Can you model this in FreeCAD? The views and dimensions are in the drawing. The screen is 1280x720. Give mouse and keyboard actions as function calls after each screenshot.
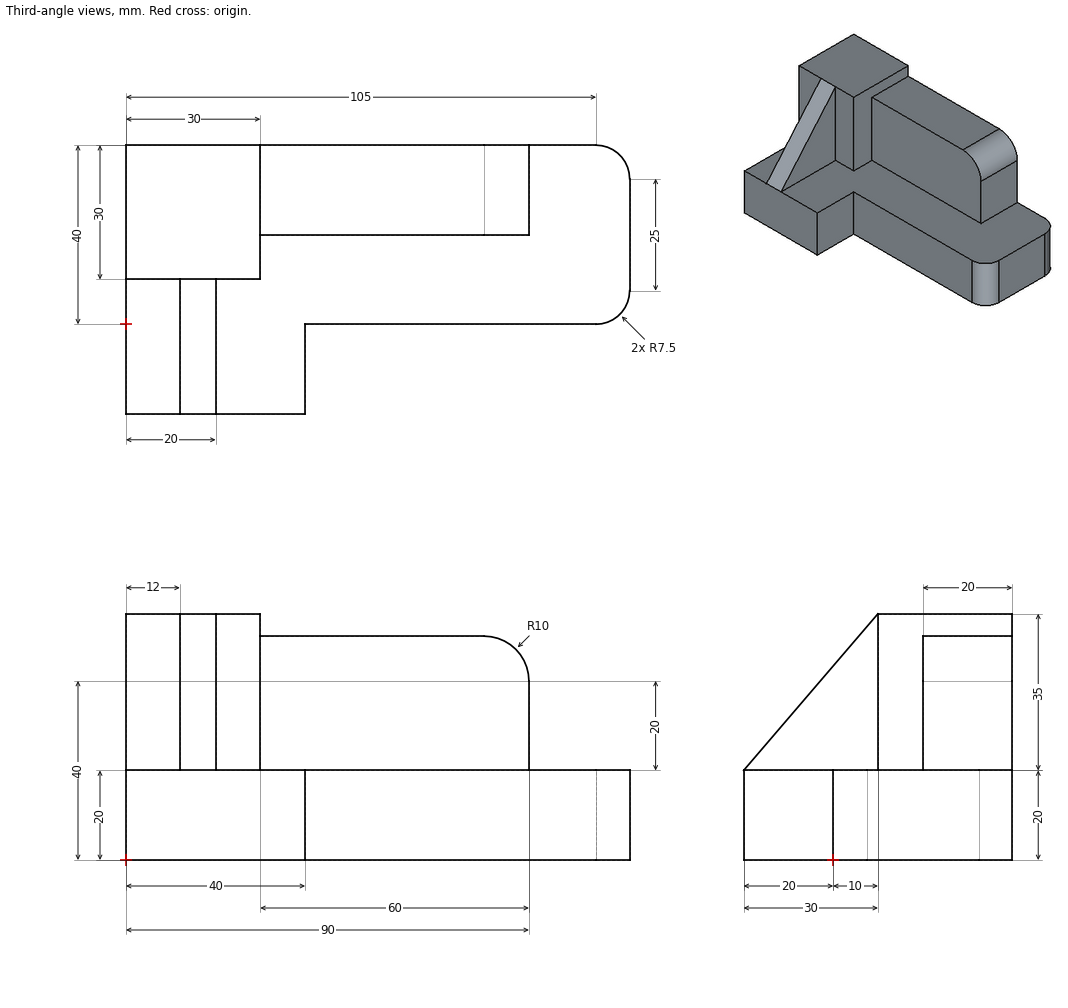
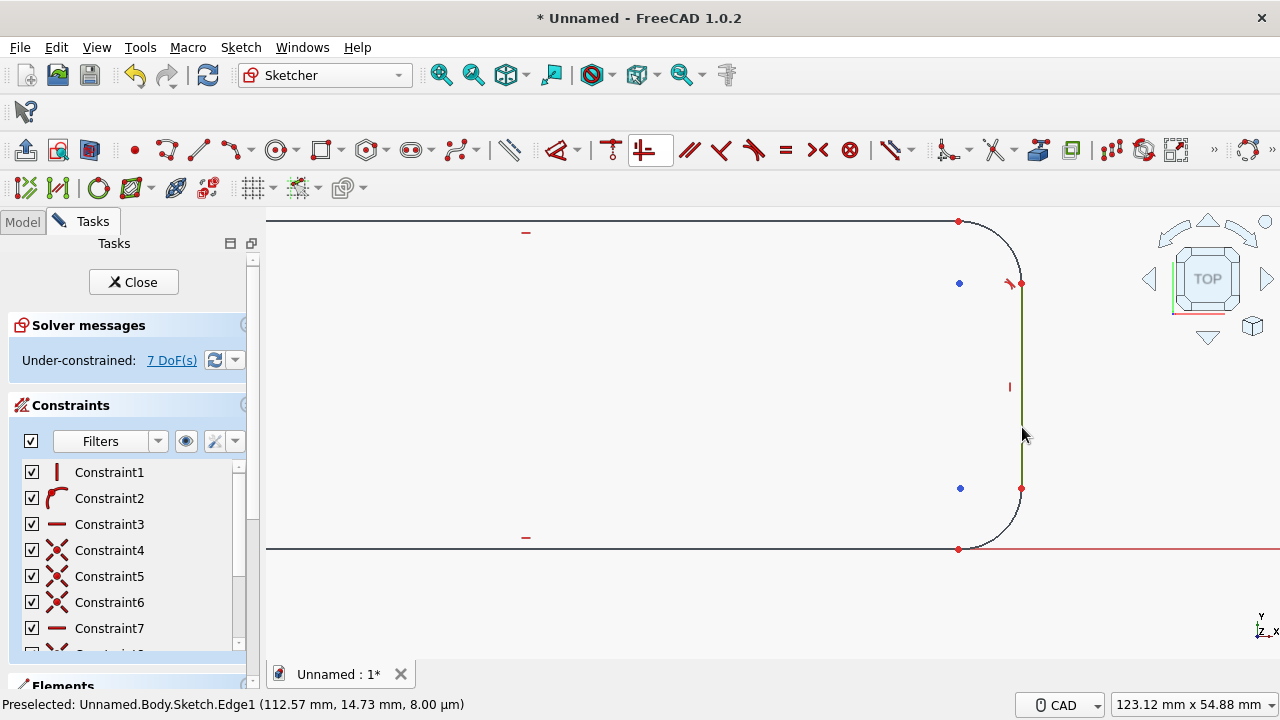
click(1015, 516)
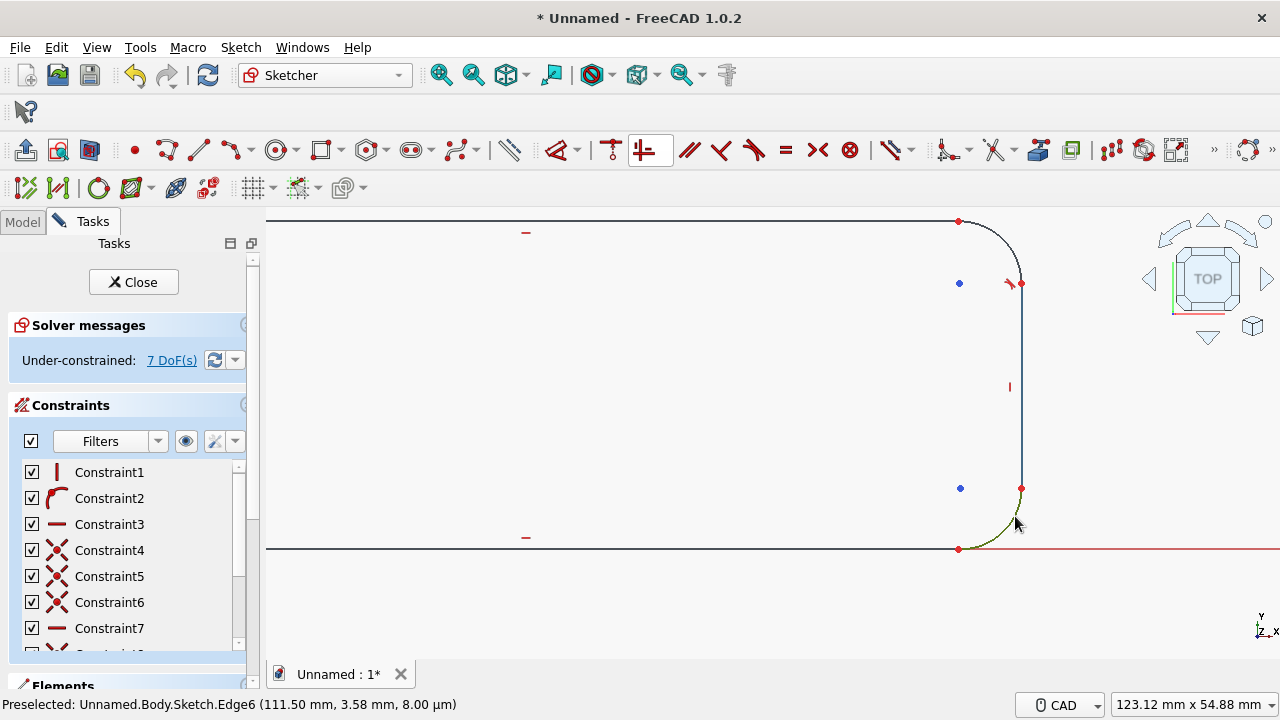
key(t)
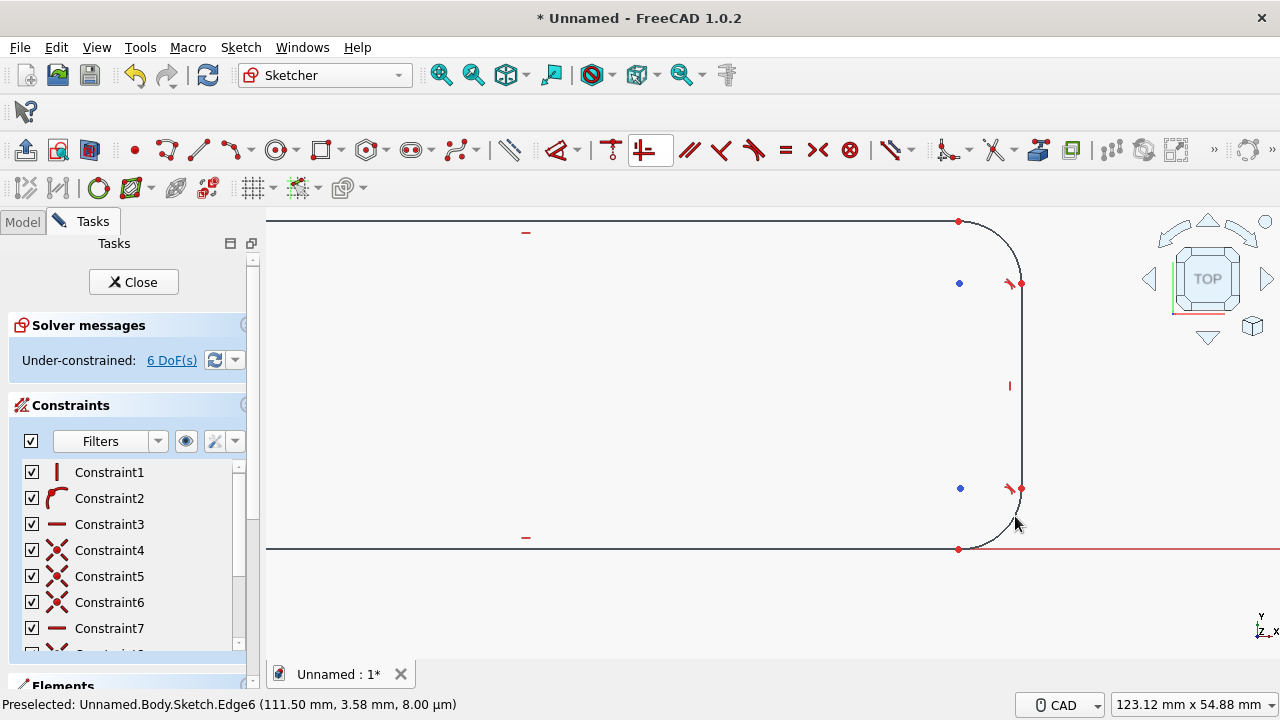
scroll(1003, 531, down, 2)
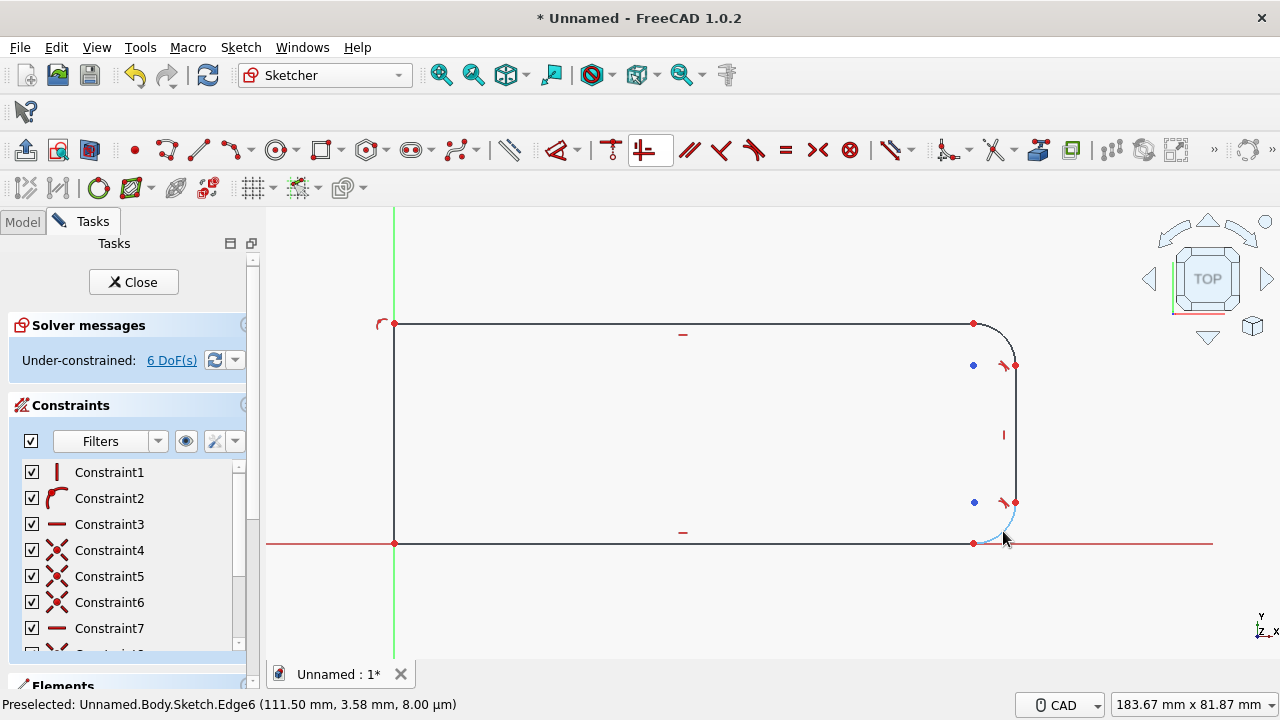
click(800, 324)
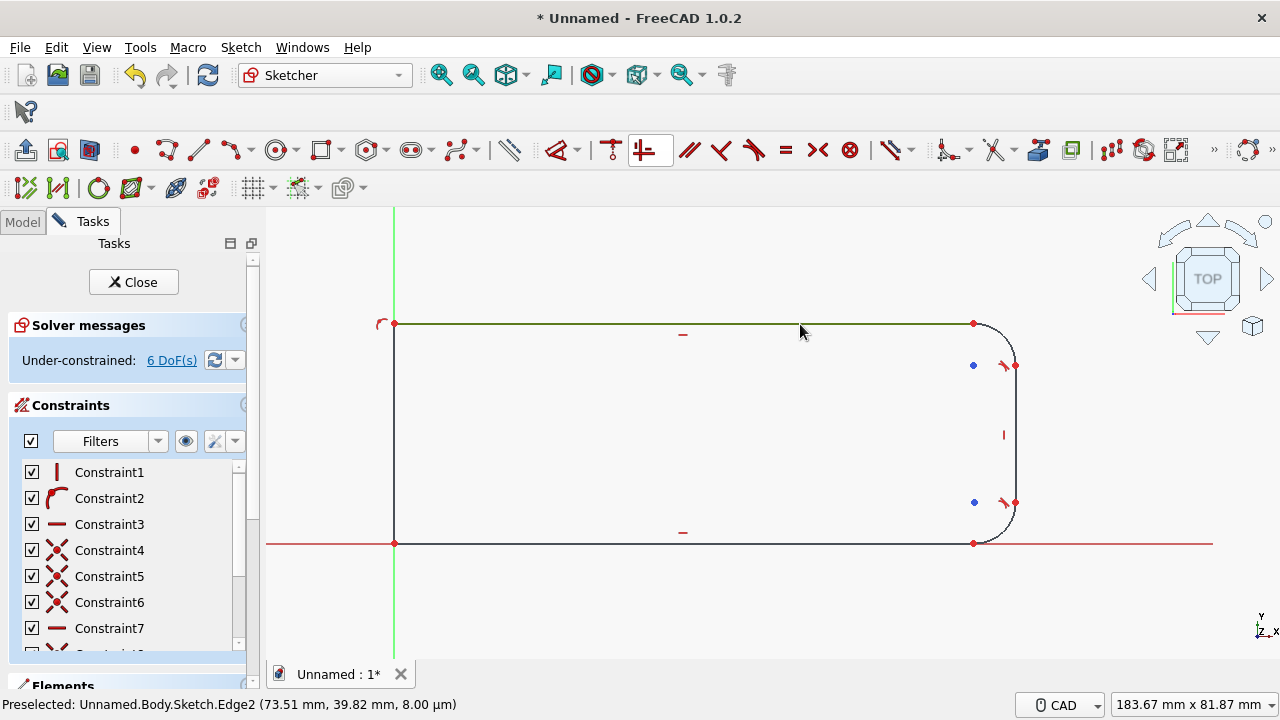
click(1011, 346)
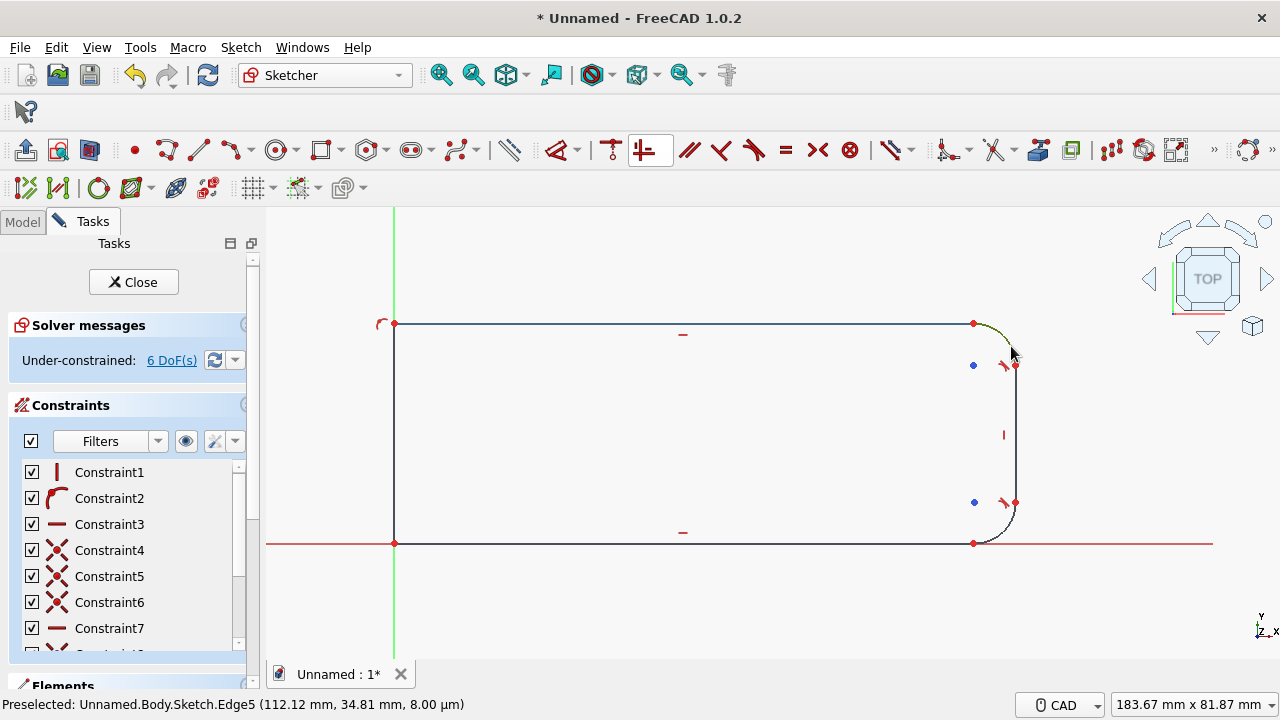
key(t)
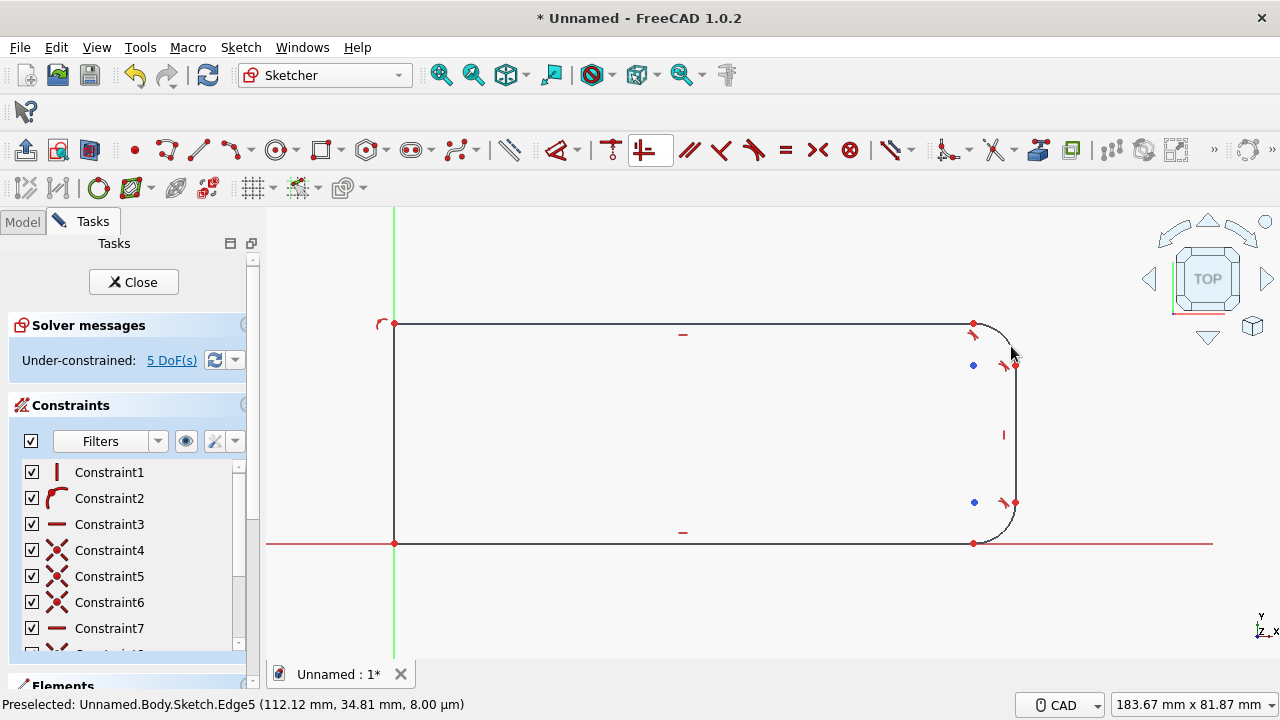
click(568, 544)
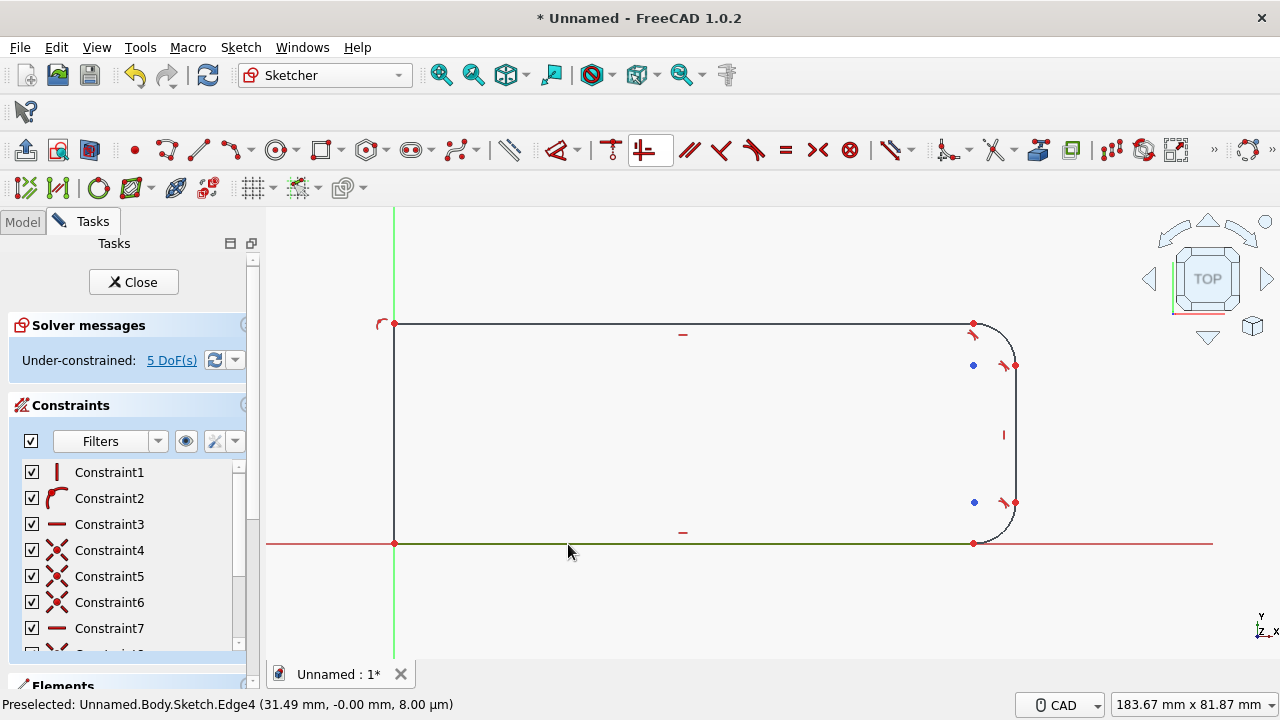
click(1011, 521)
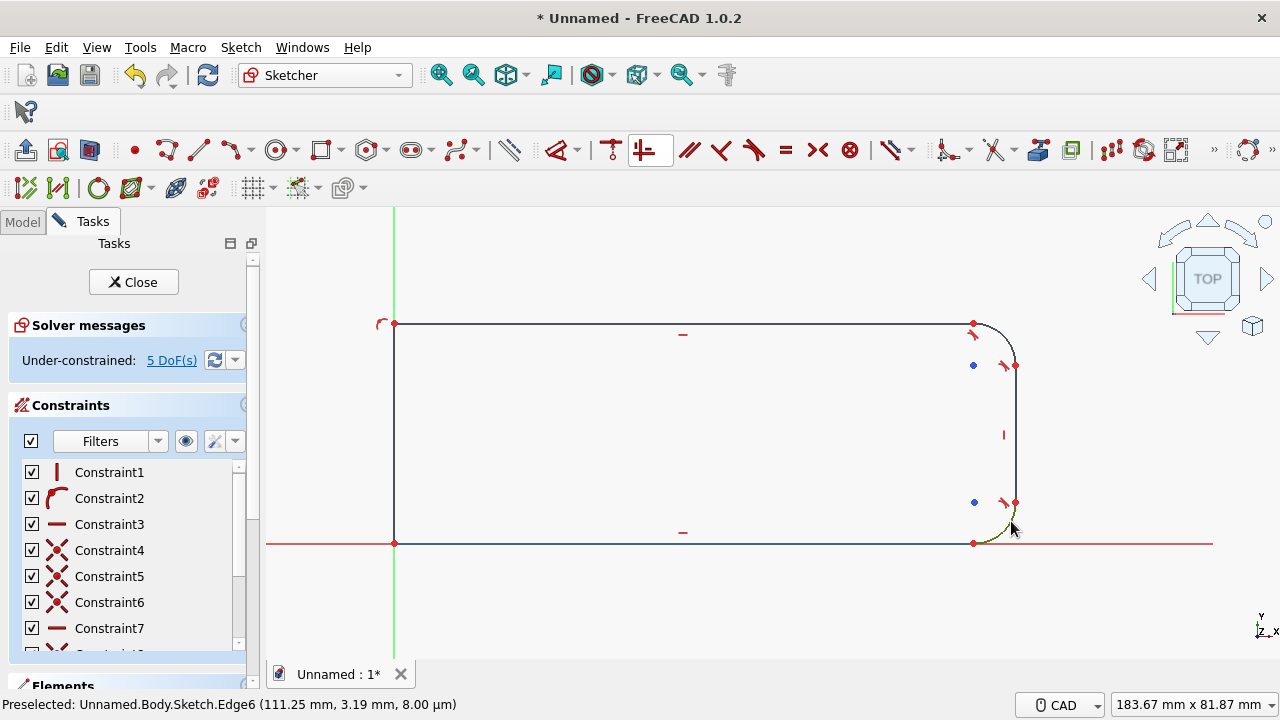
key(t)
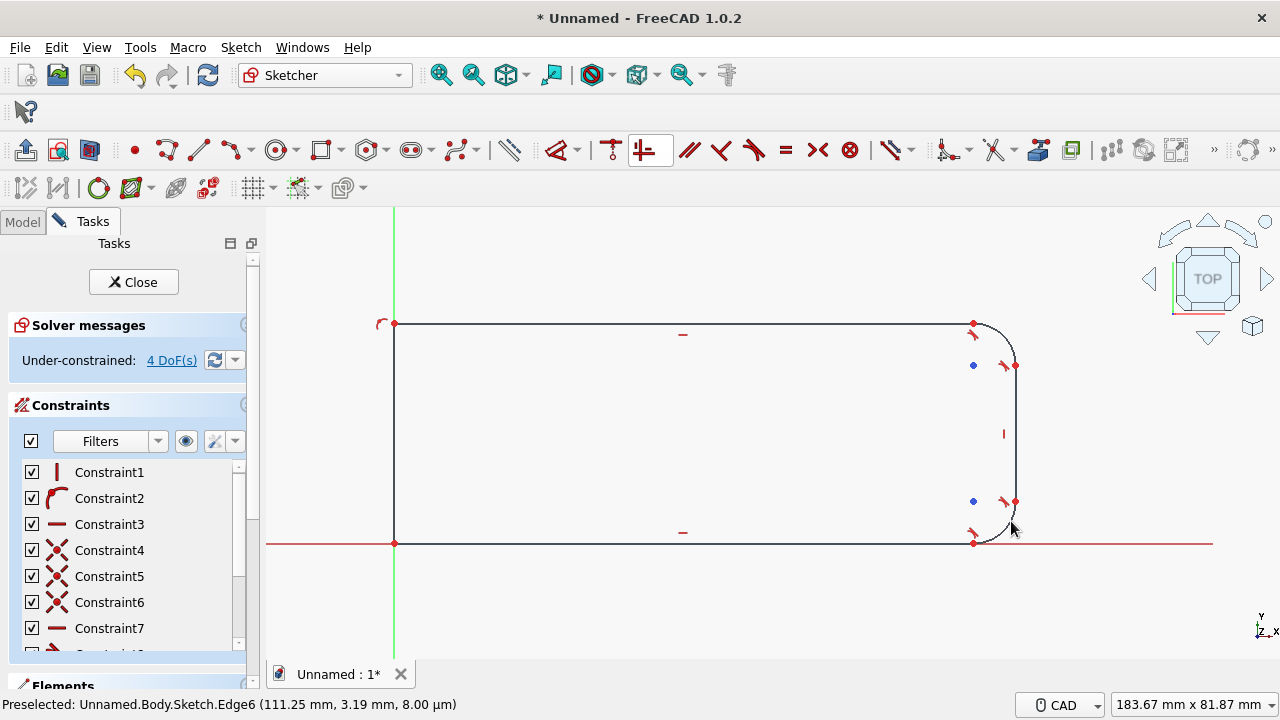
click(1011, 346)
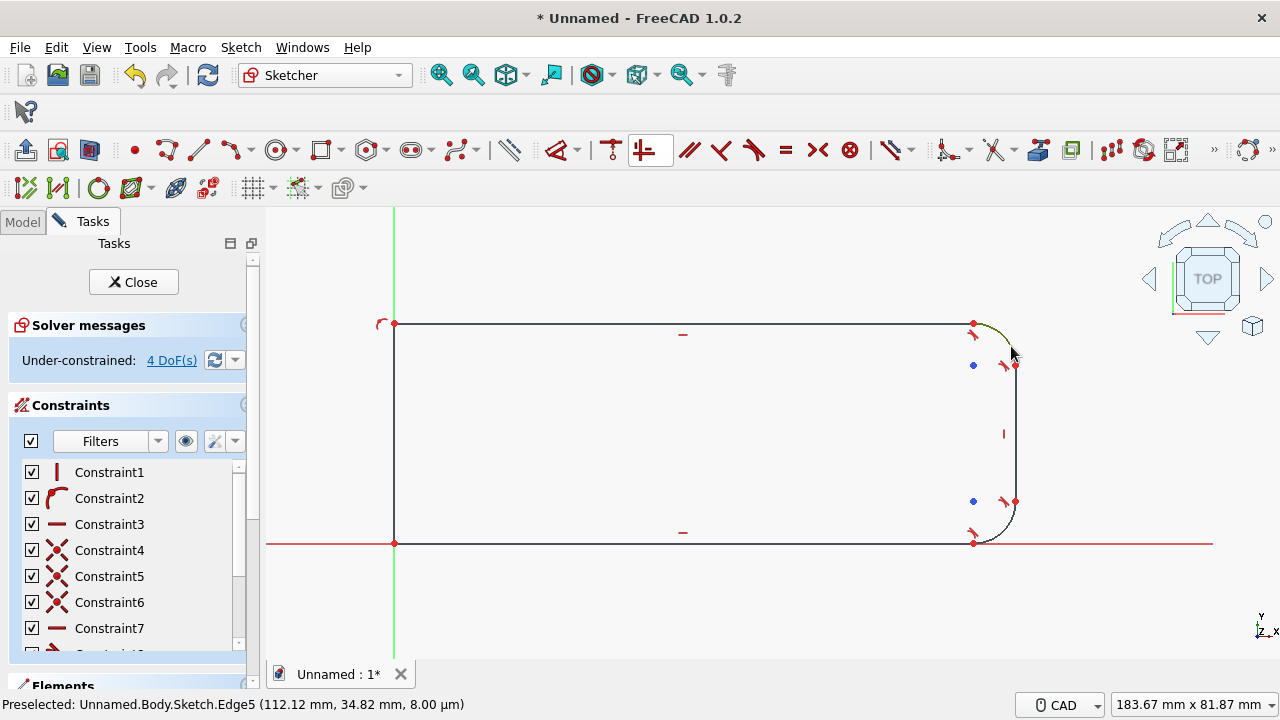
click(1011, 521)